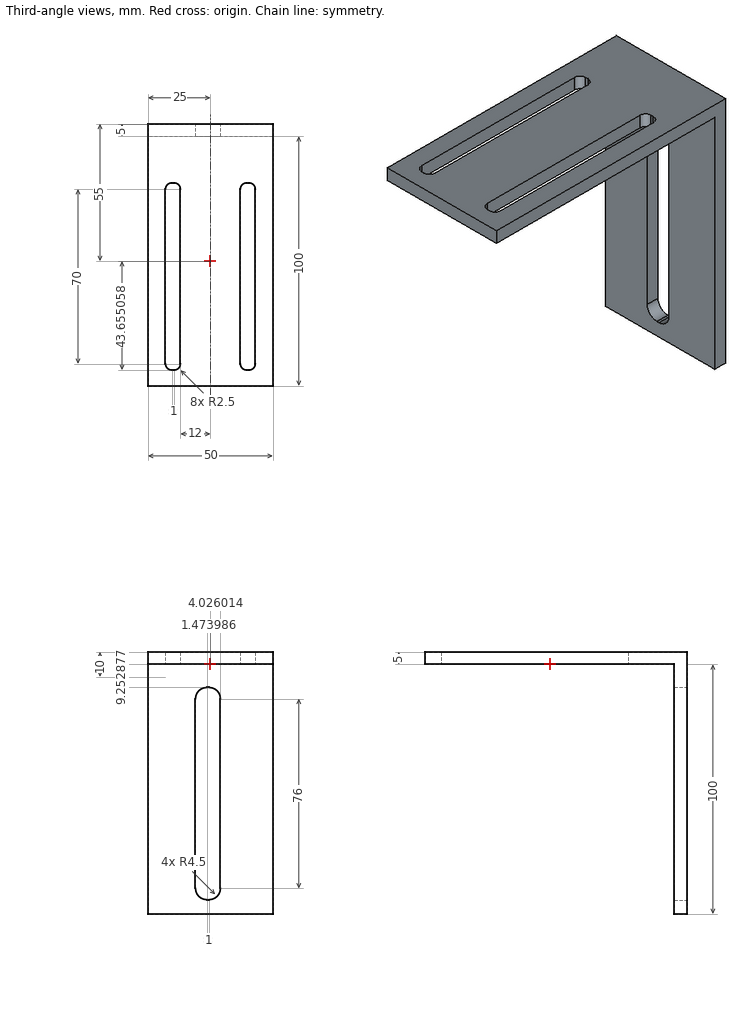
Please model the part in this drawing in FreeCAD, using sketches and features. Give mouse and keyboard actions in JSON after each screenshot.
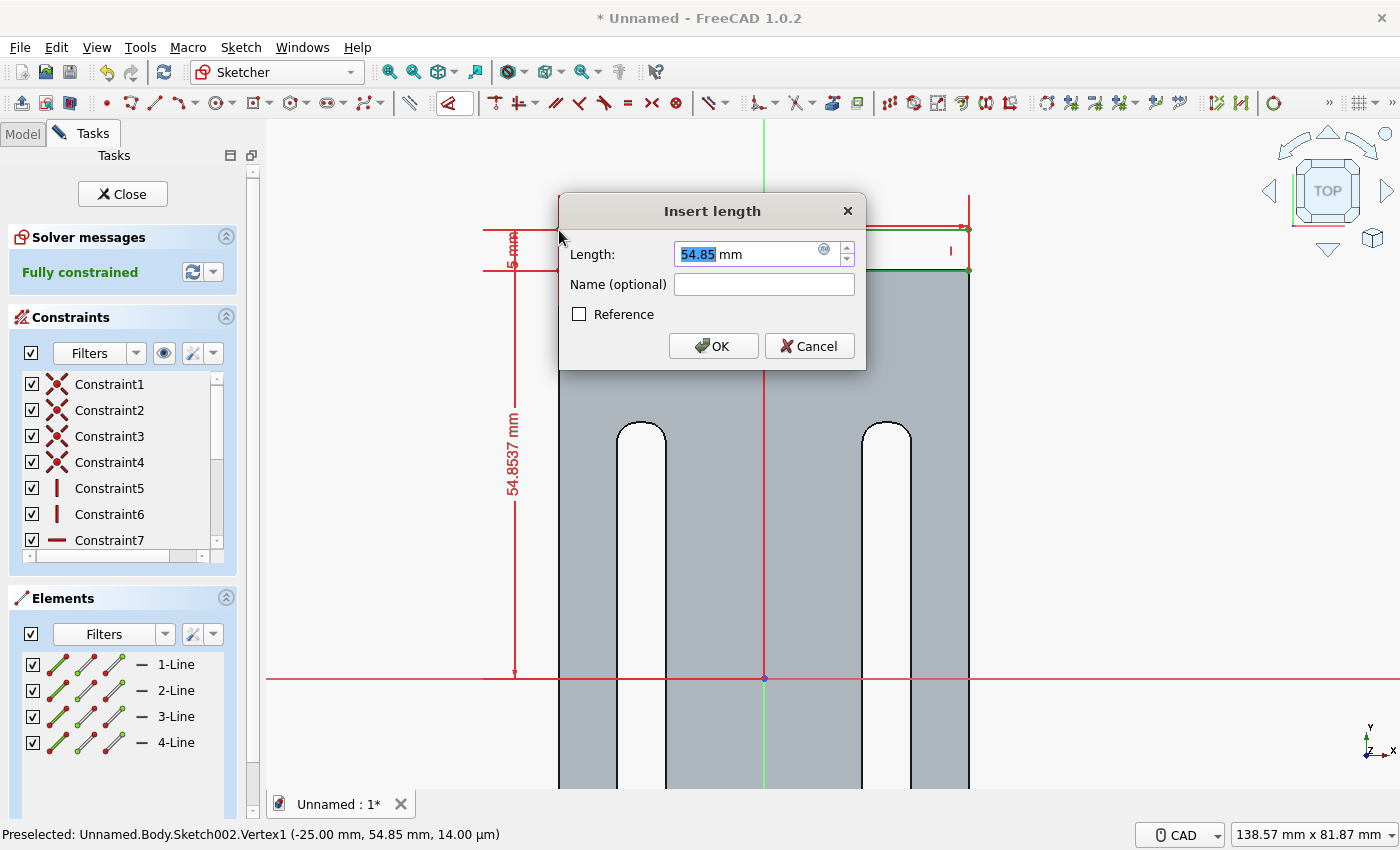
{"action": "type", "text": "55"}
{"action": "key", "text": "Return"}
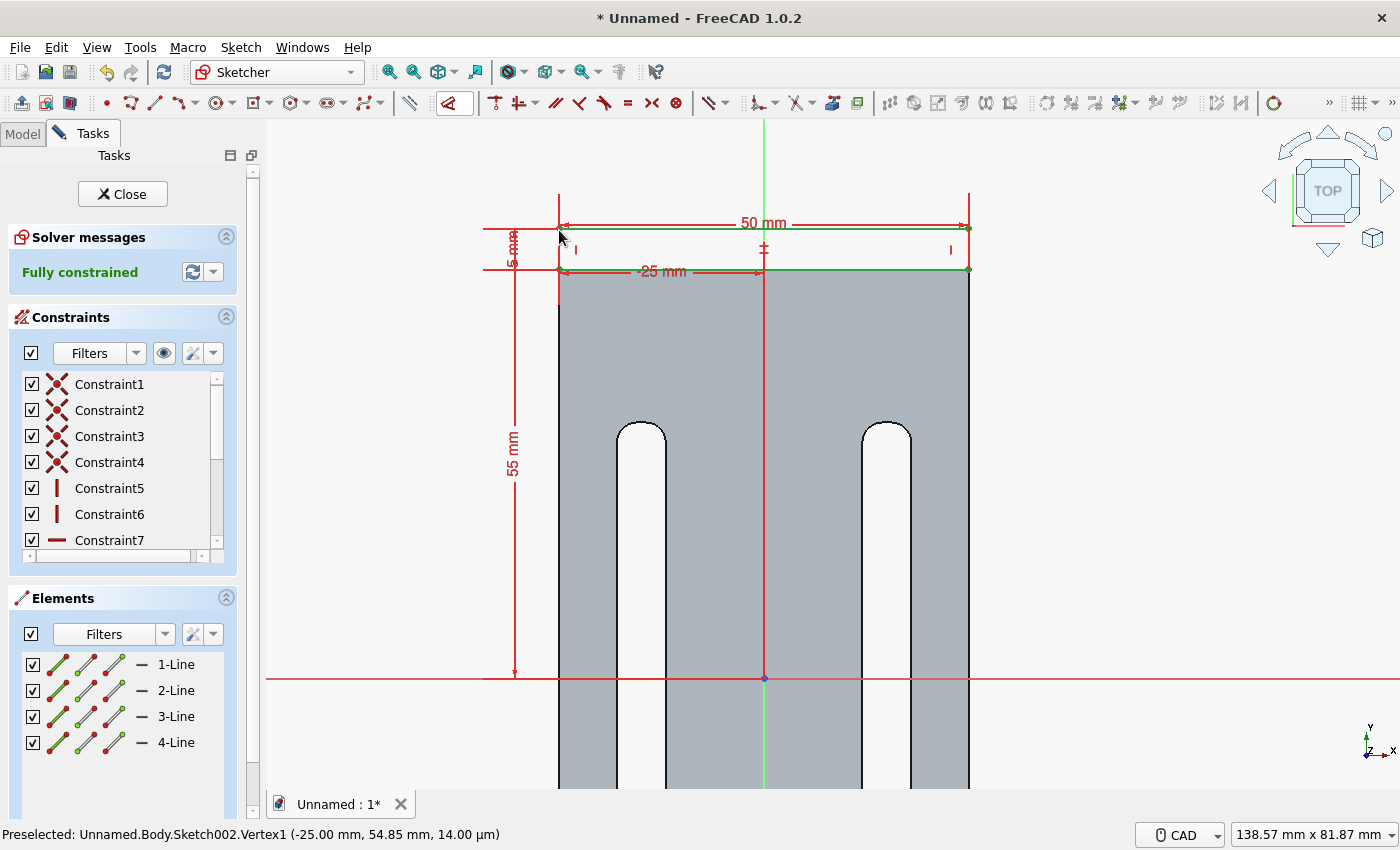
{"action": "left_click", "coordinate": [123, 194]}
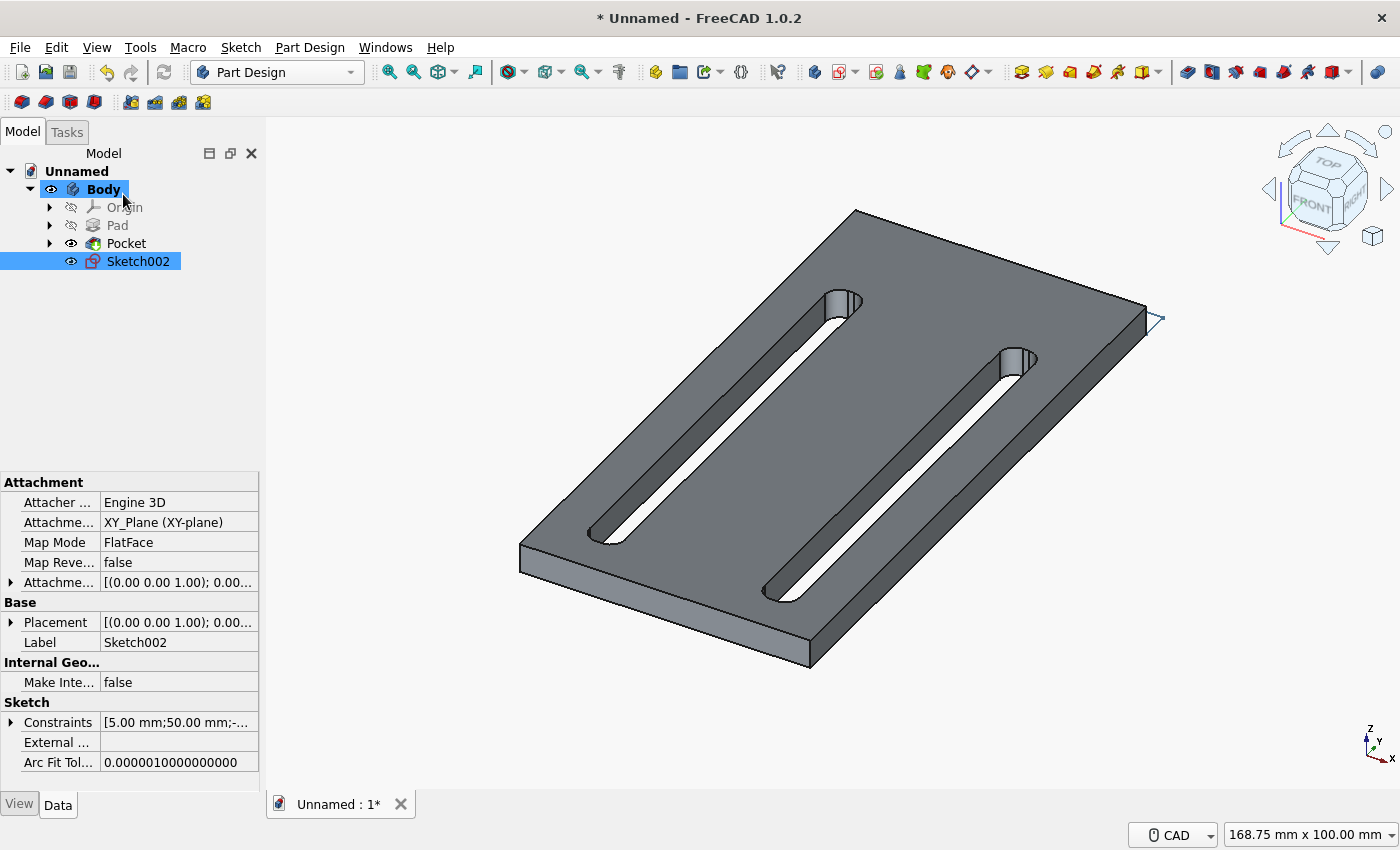
{"action": "left_click", "coordinate": [1022, 72]}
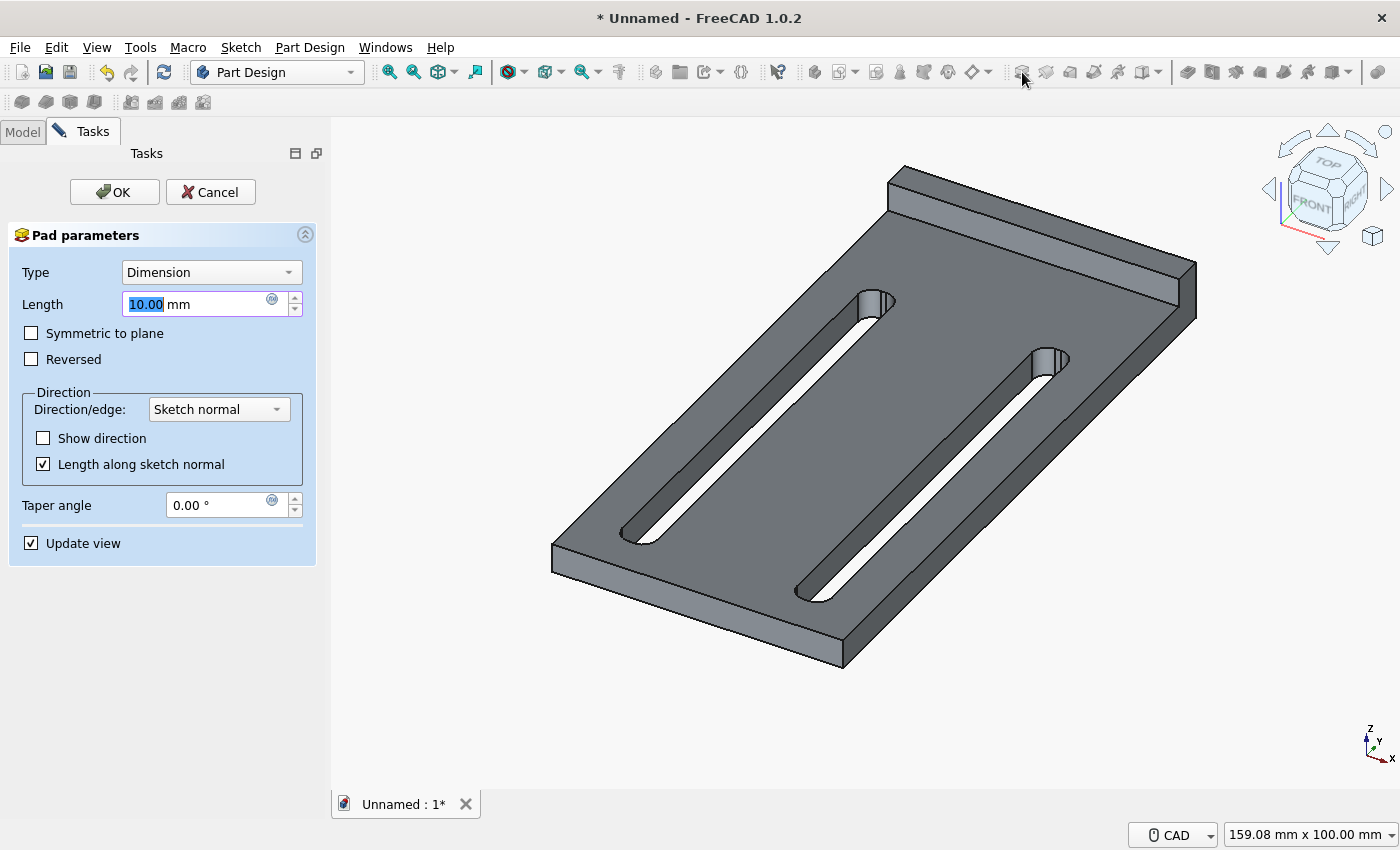
{"action": "left_click", "coordinate": [212, 272]}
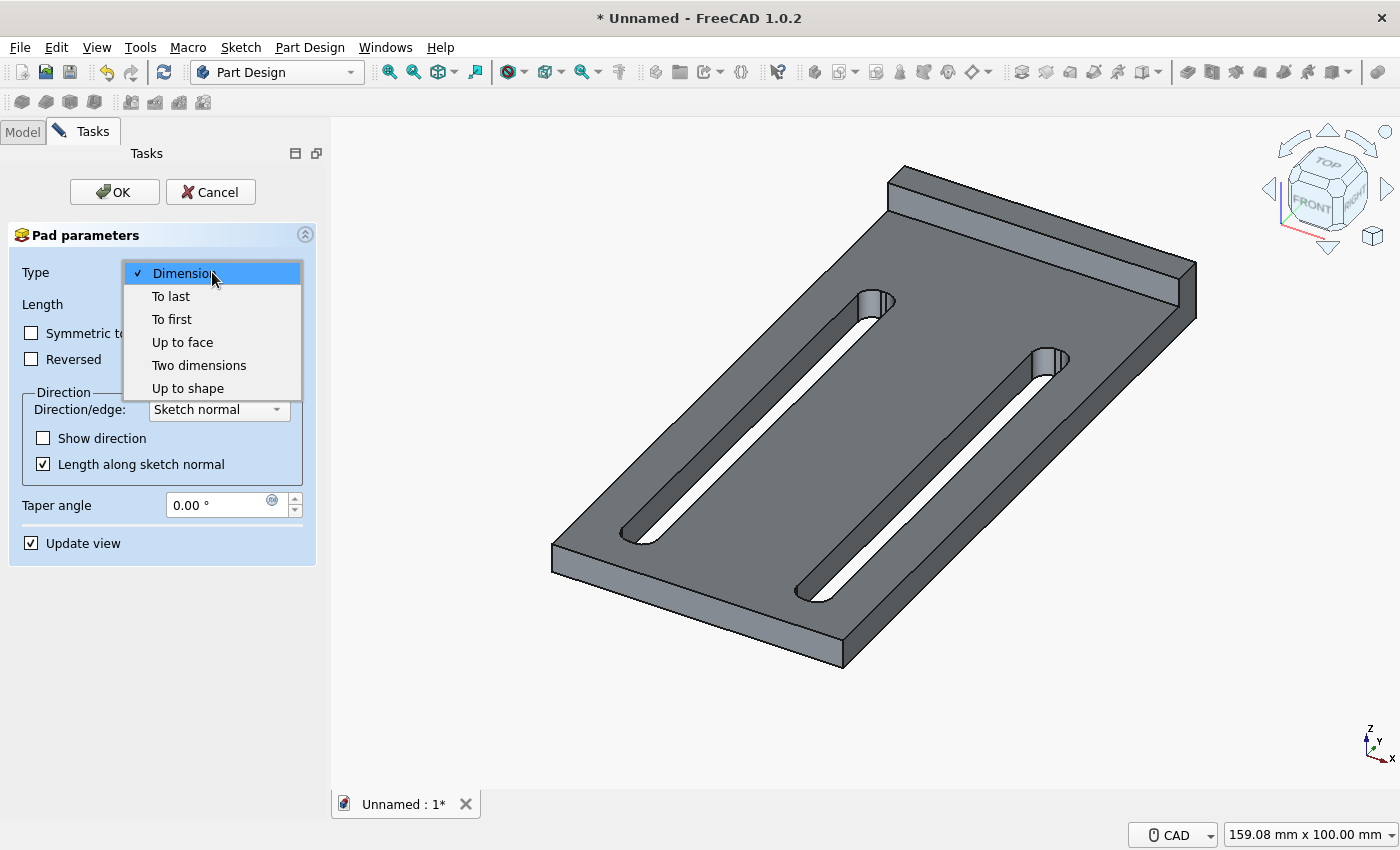
{"action": "left_click", "coordinate": [212, 366]}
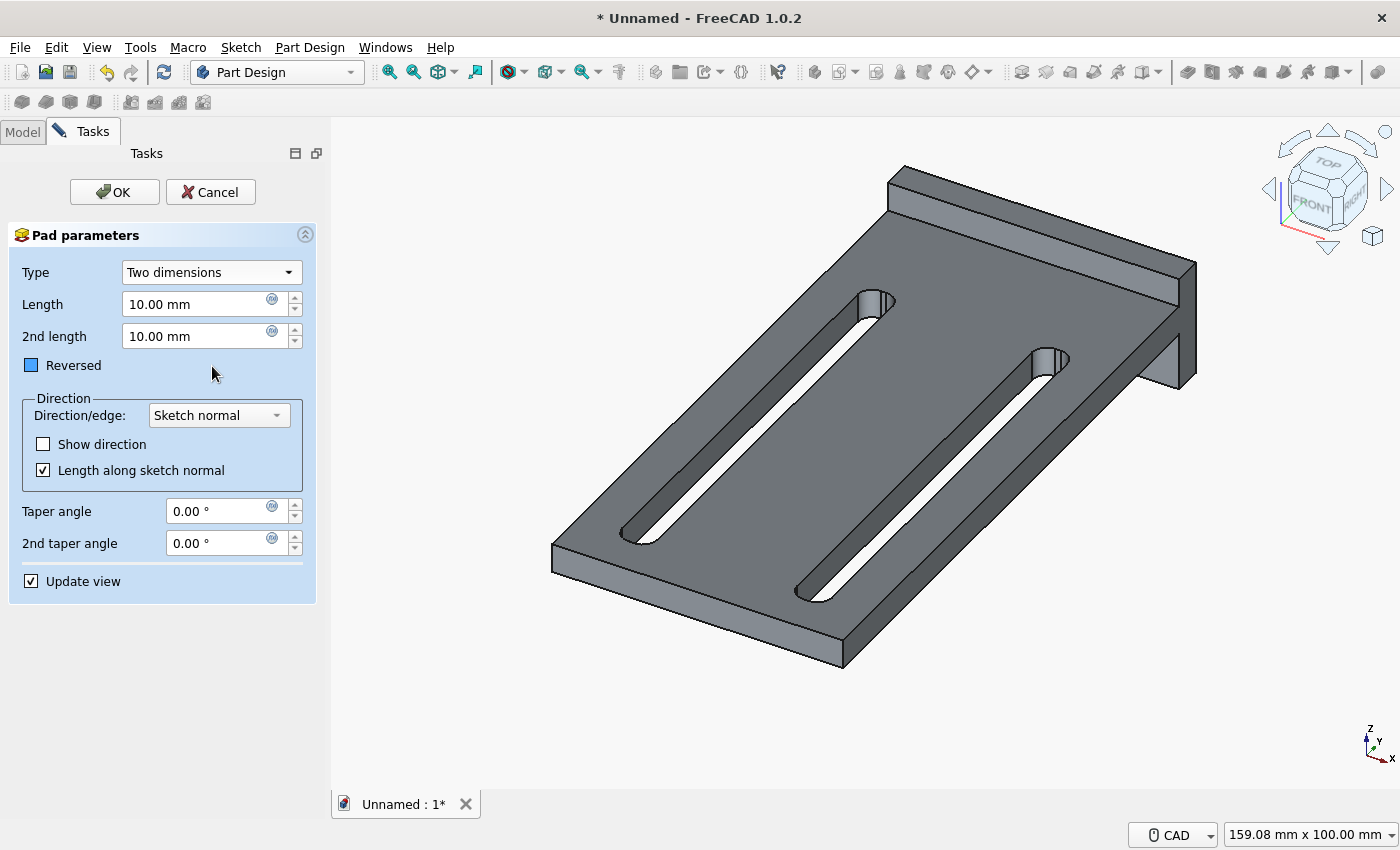
{"action": "triple_click", "coordinate": [204, 304]}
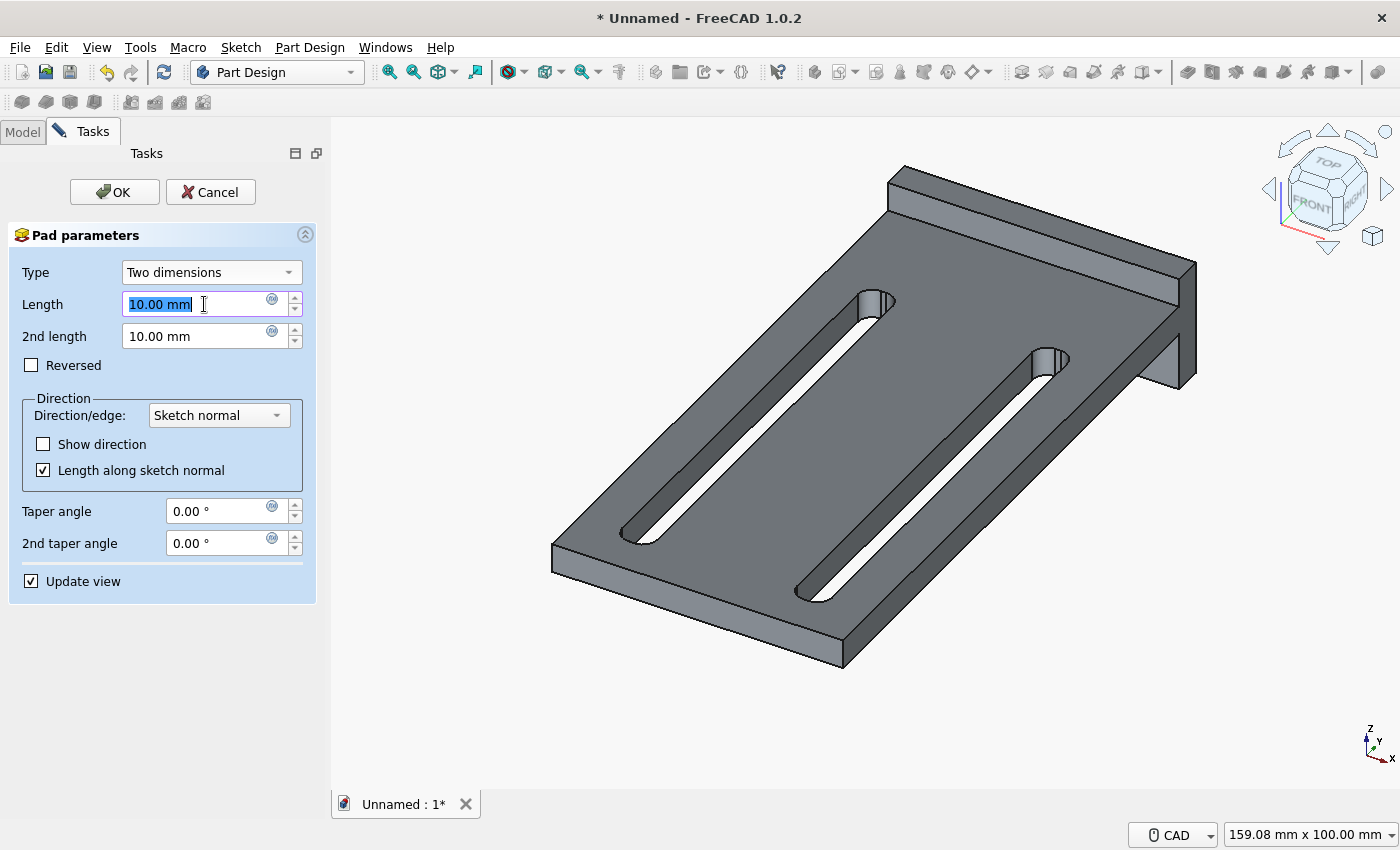
{"action": "type", "text": "100"}
{"action": "key", "text": "Tab"}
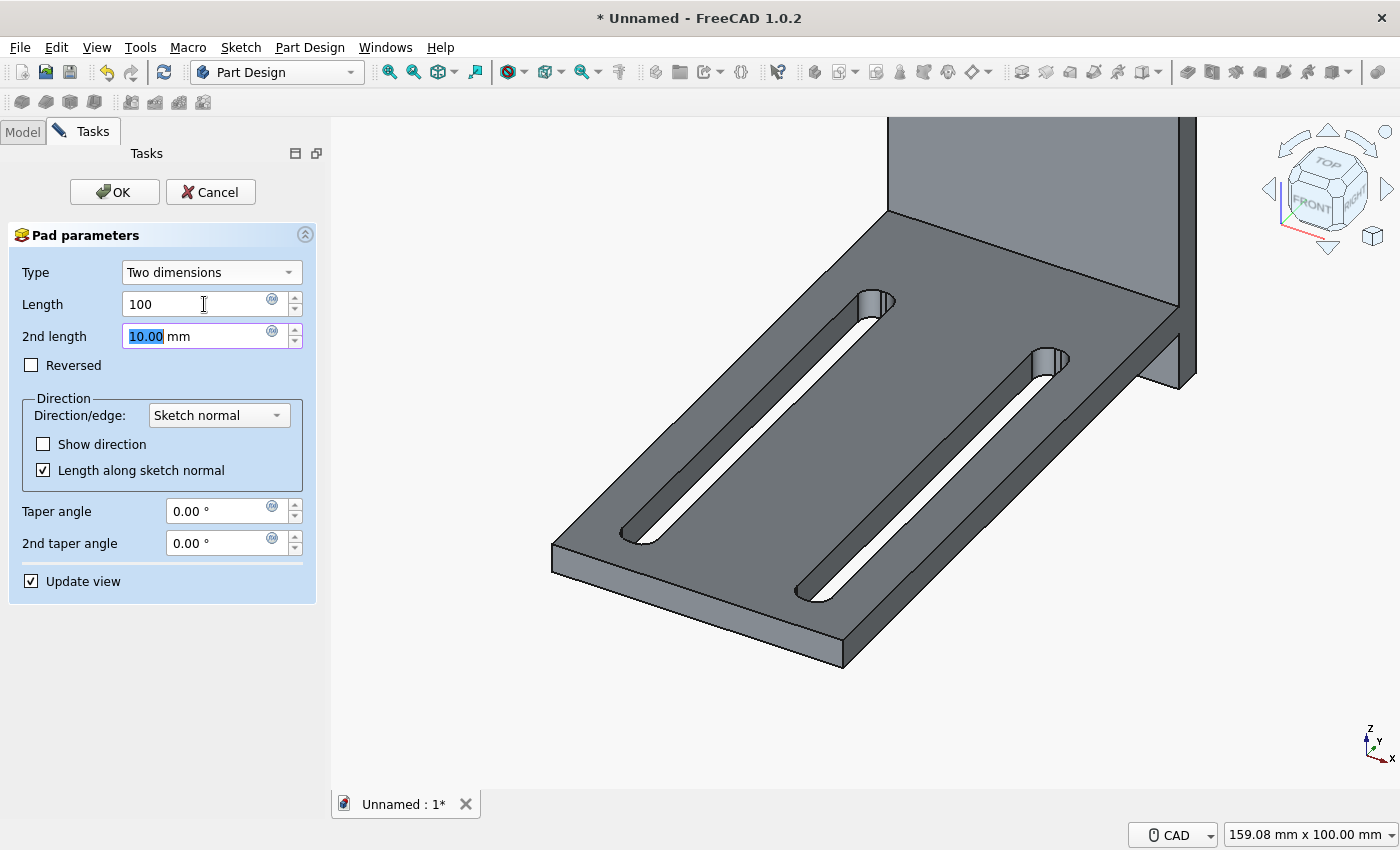
{"action": "type", "text": "5"}
{"action": "key", "text": "Tab"}